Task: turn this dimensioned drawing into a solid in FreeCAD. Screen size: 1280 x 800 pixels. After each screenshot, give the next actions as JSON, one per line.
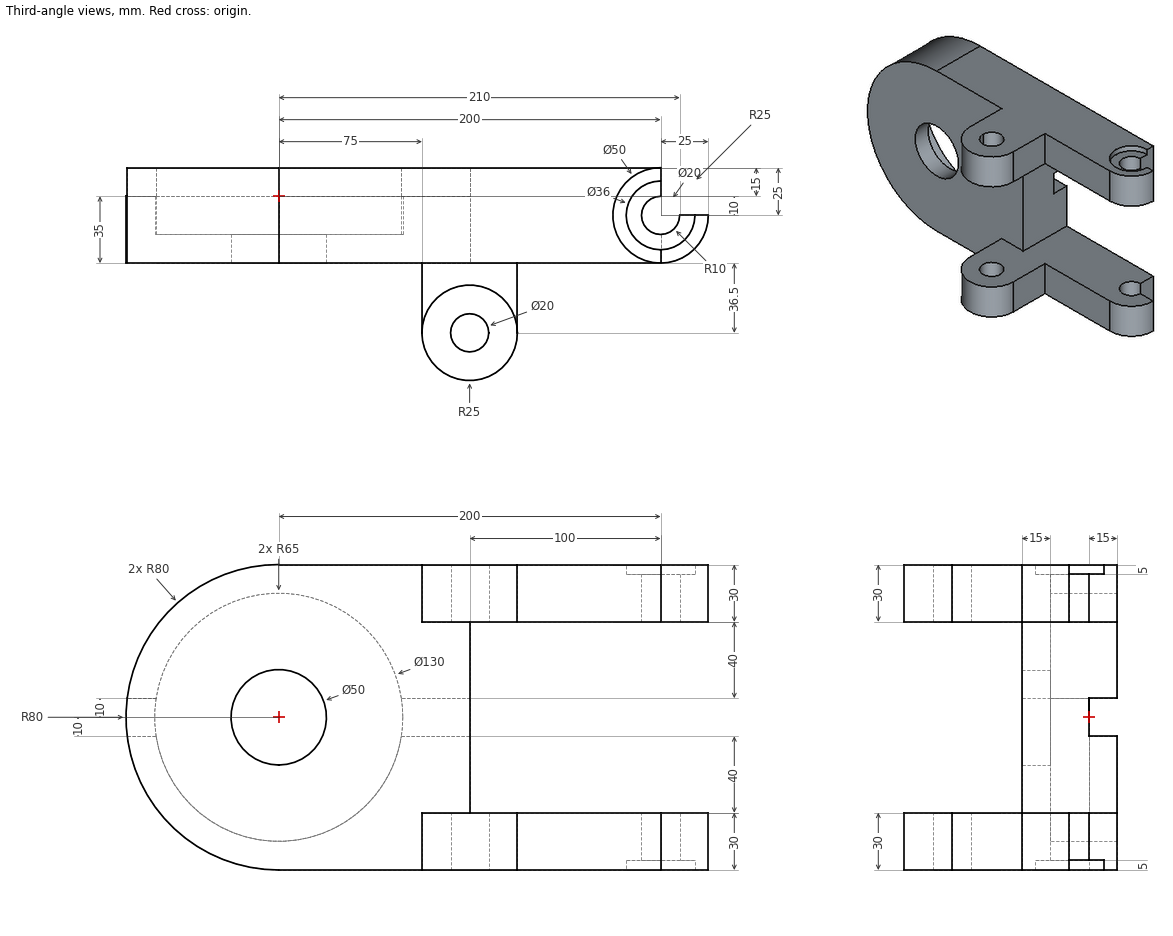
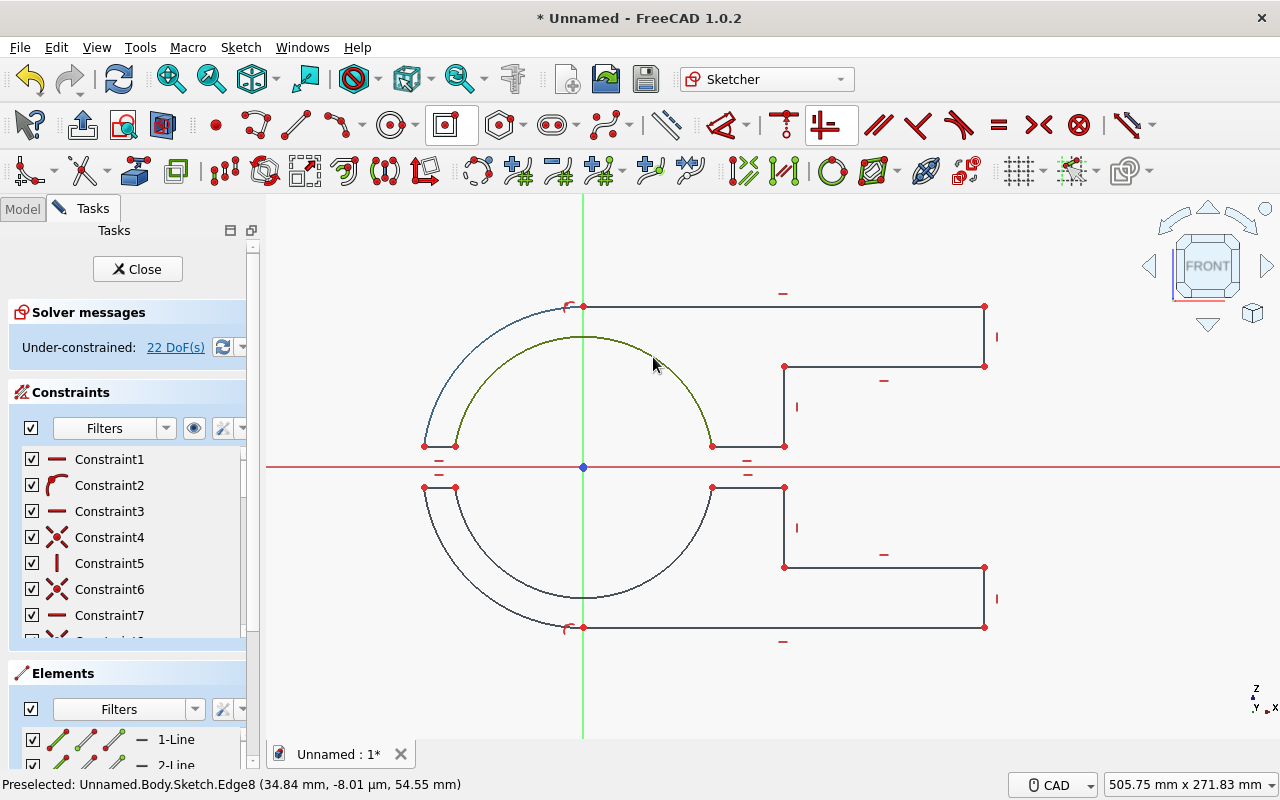
{"action": "left_click", "coordinate": [784, 126]}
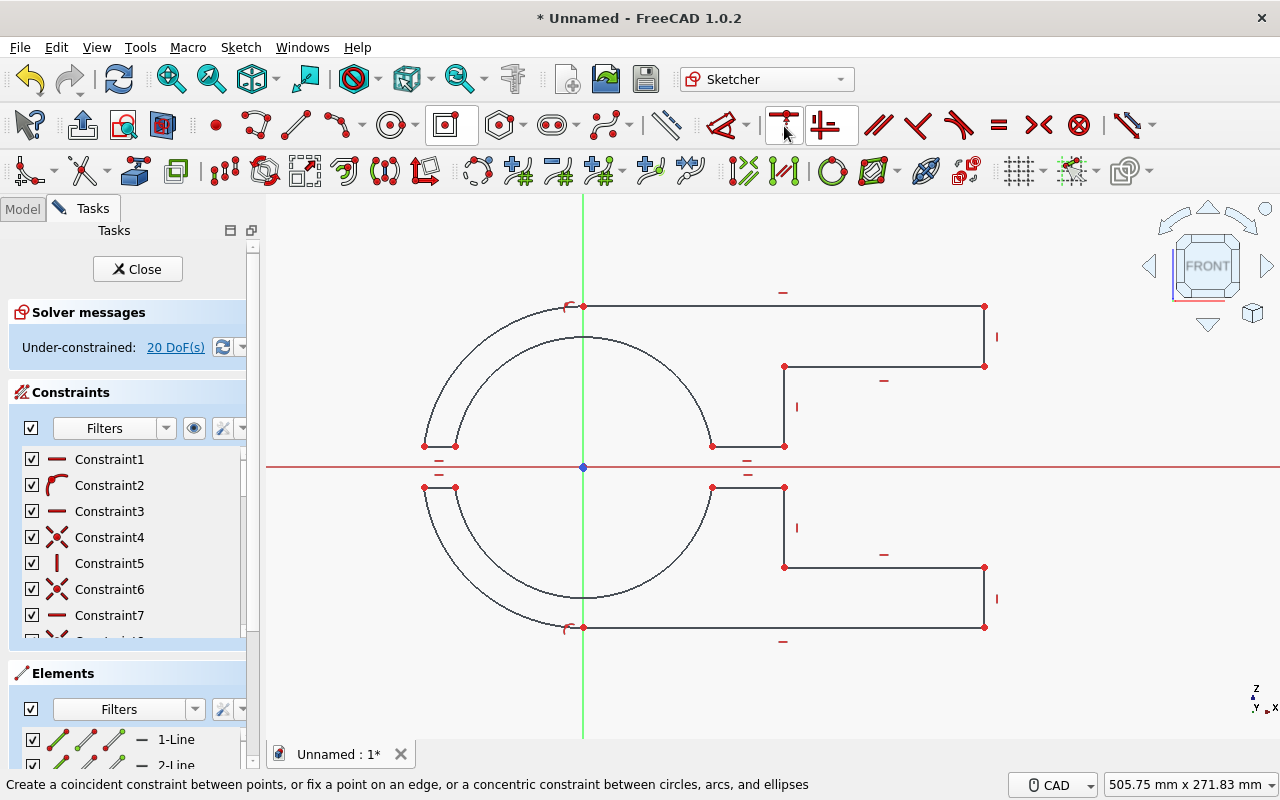
{"action": "left_click", "coordinate": [516, 321]}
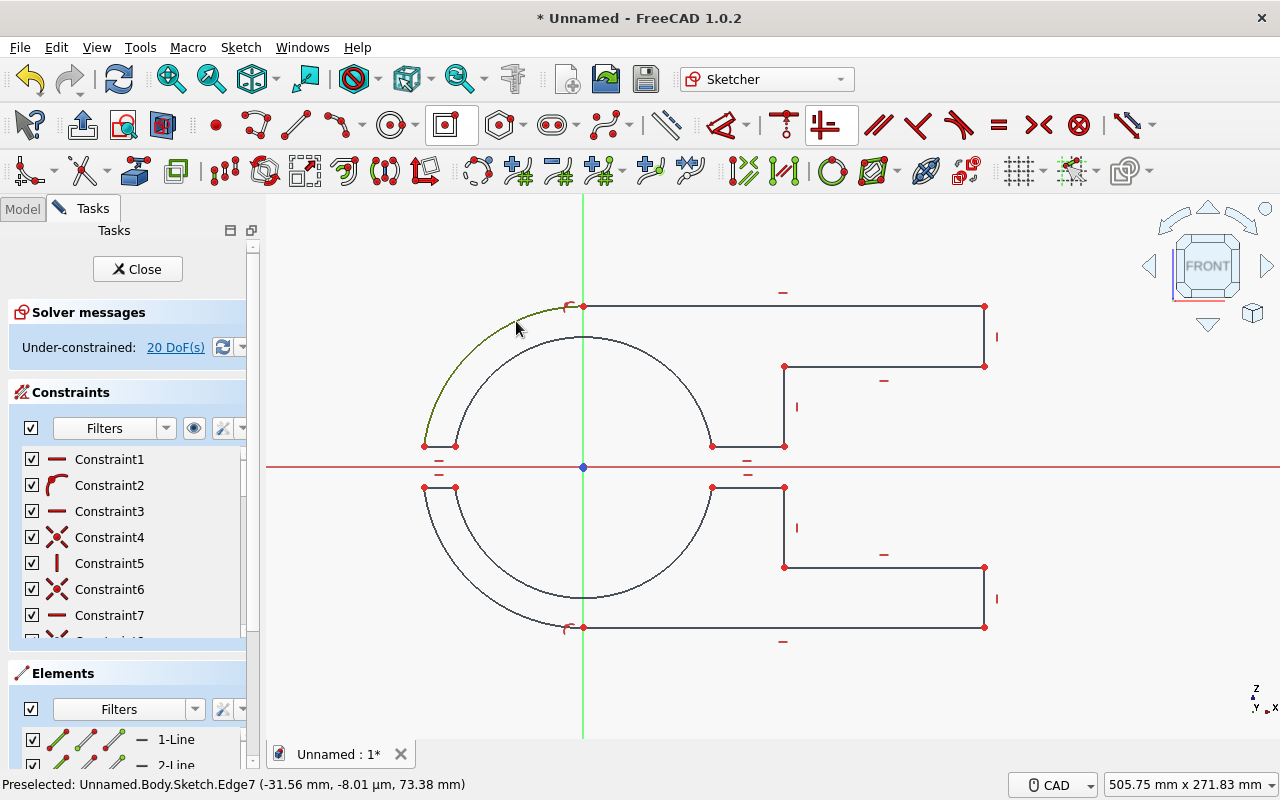
{"action": "left_click", "coordinate": [514, 578]}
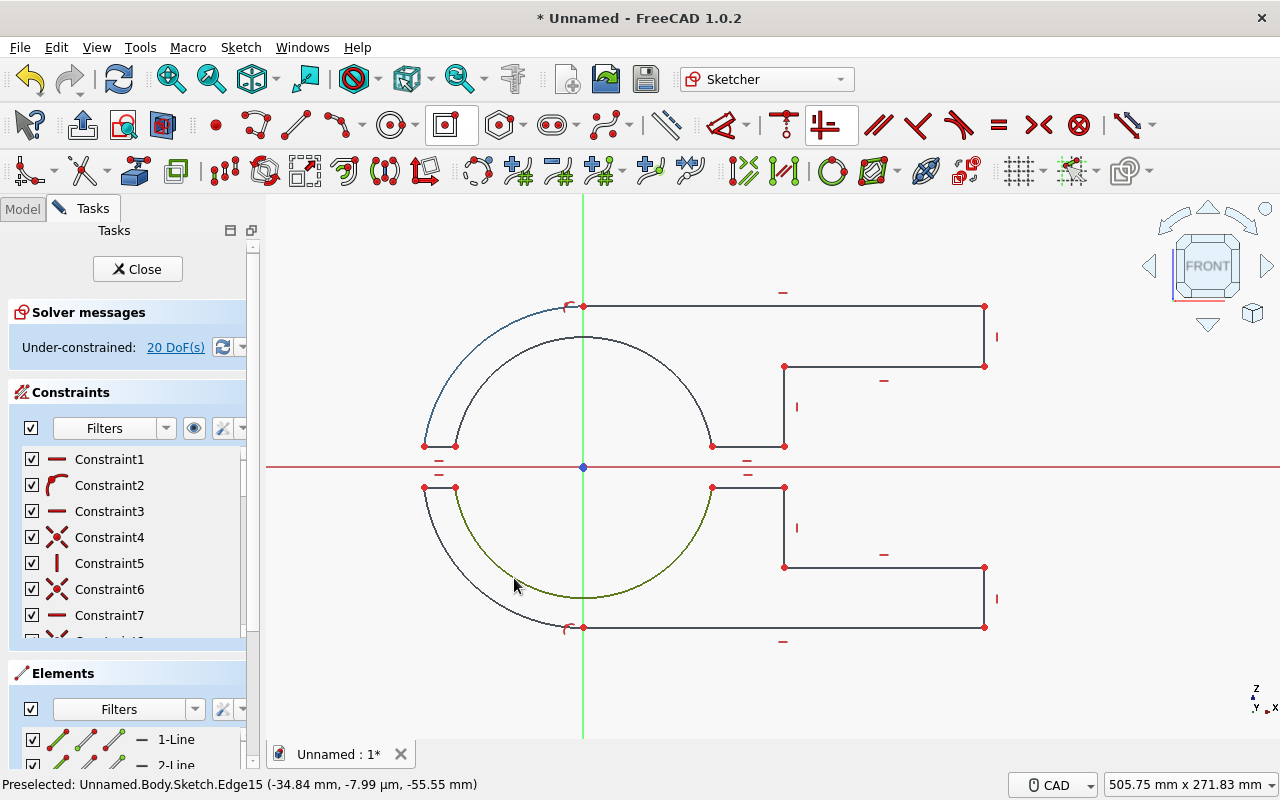
{"action": "left_click", "coordinate": [784, 126]}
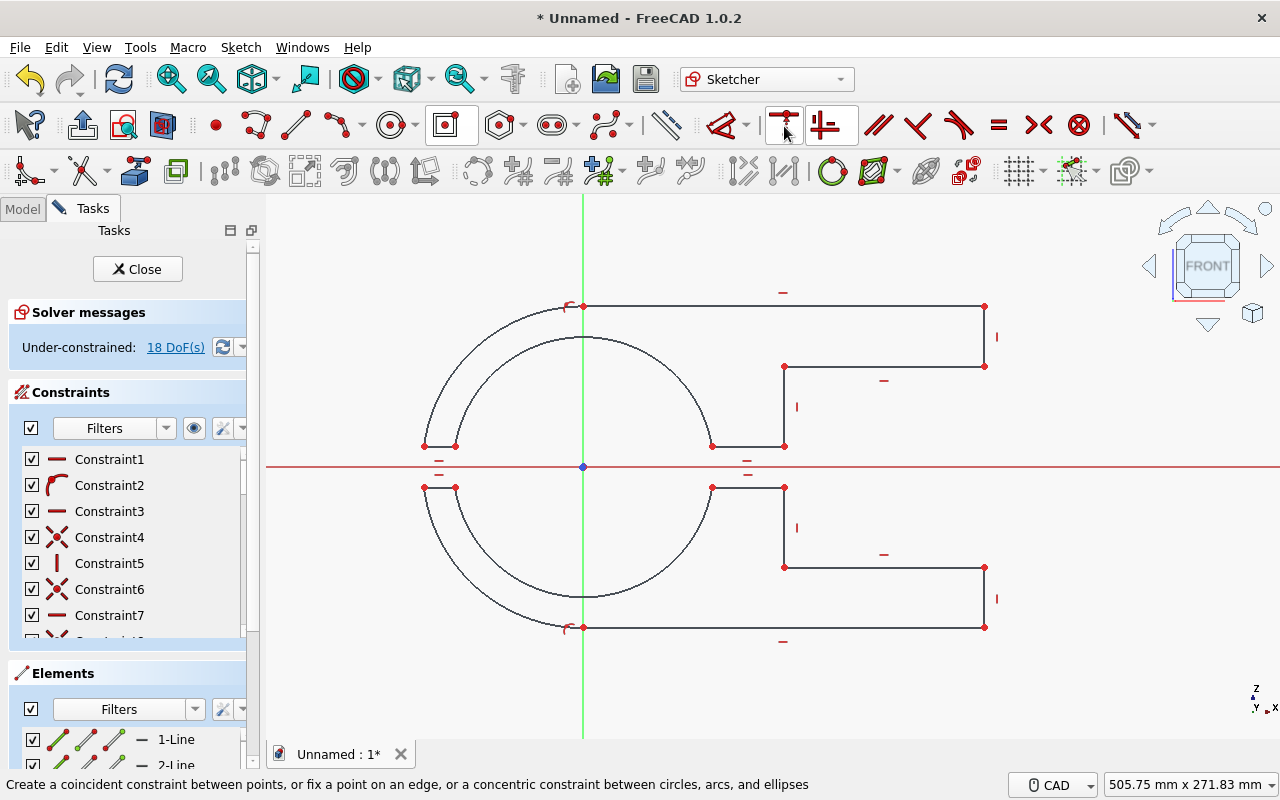
{"action": "left_click", "coordinate": [516, 321]}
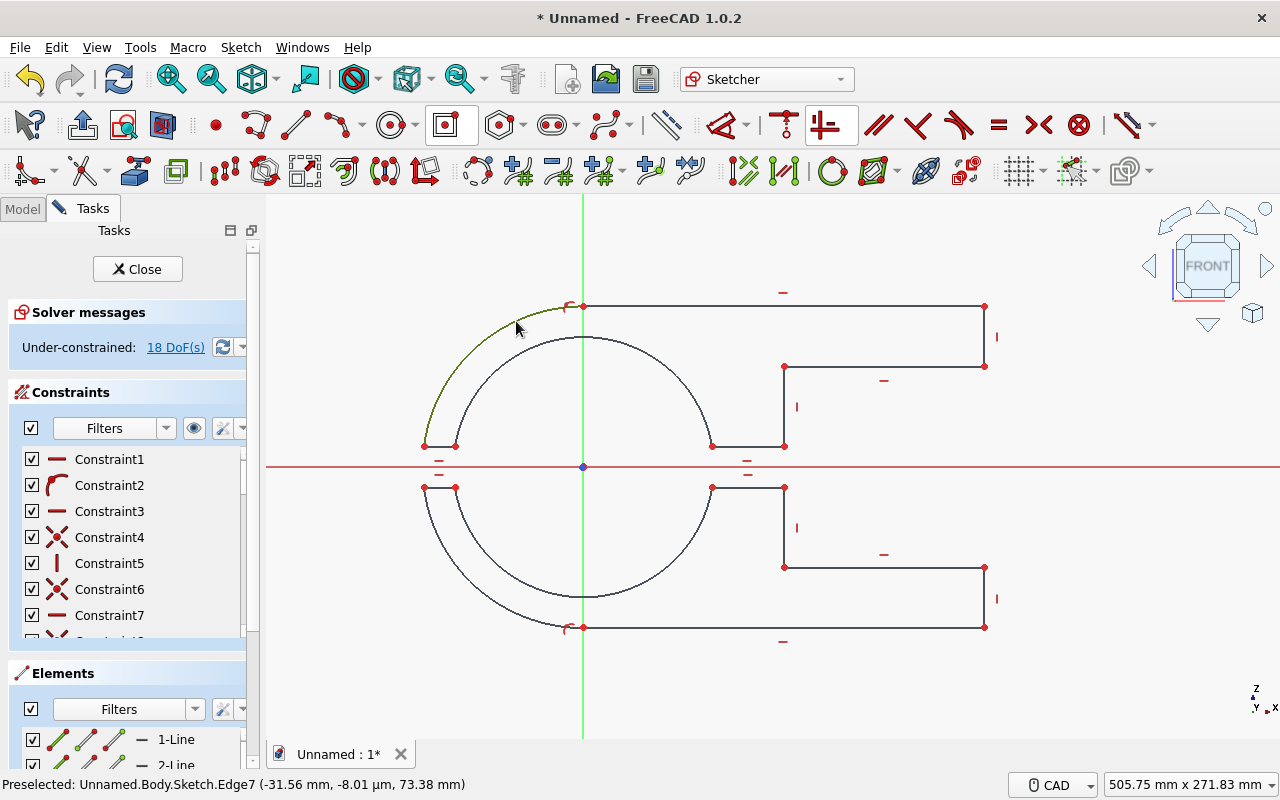
{"action": "left_click", "coordinate": [447, 553]}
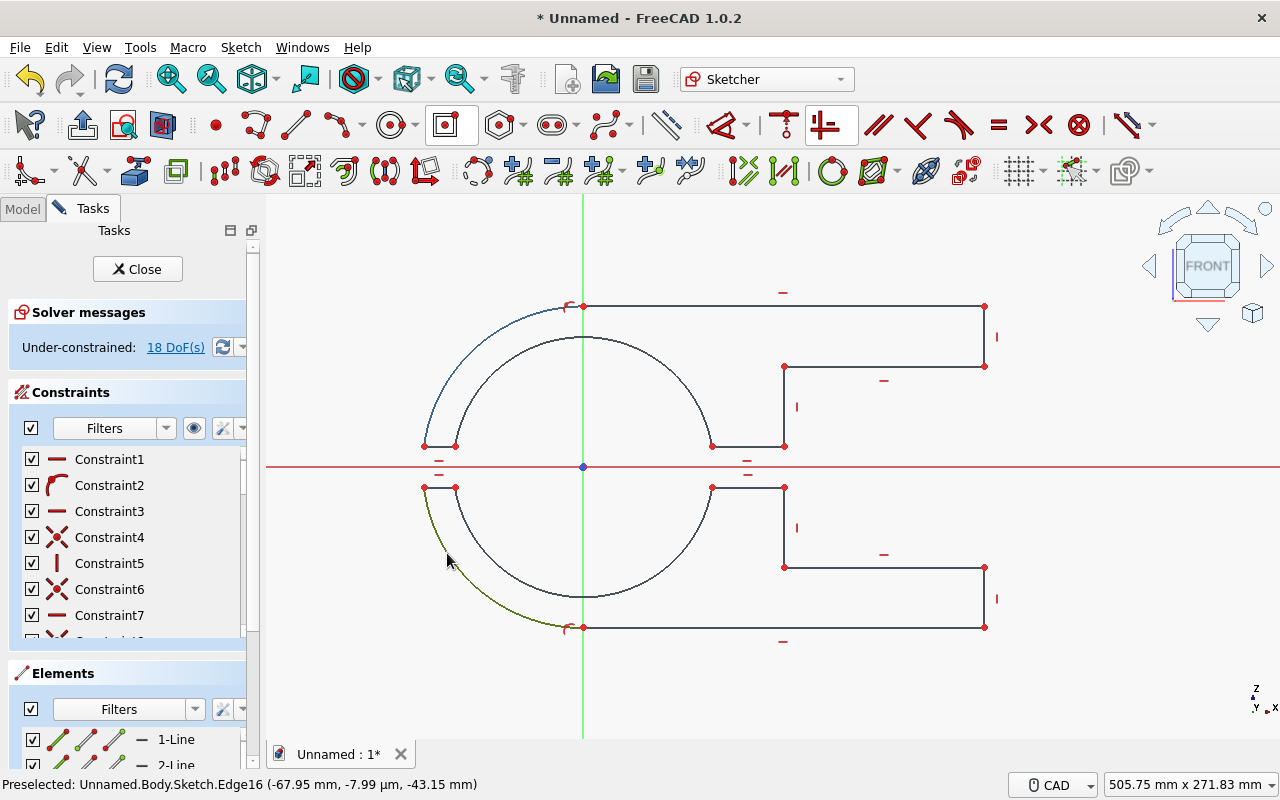
{"action": "left_click", "coordinate": [784, 126]}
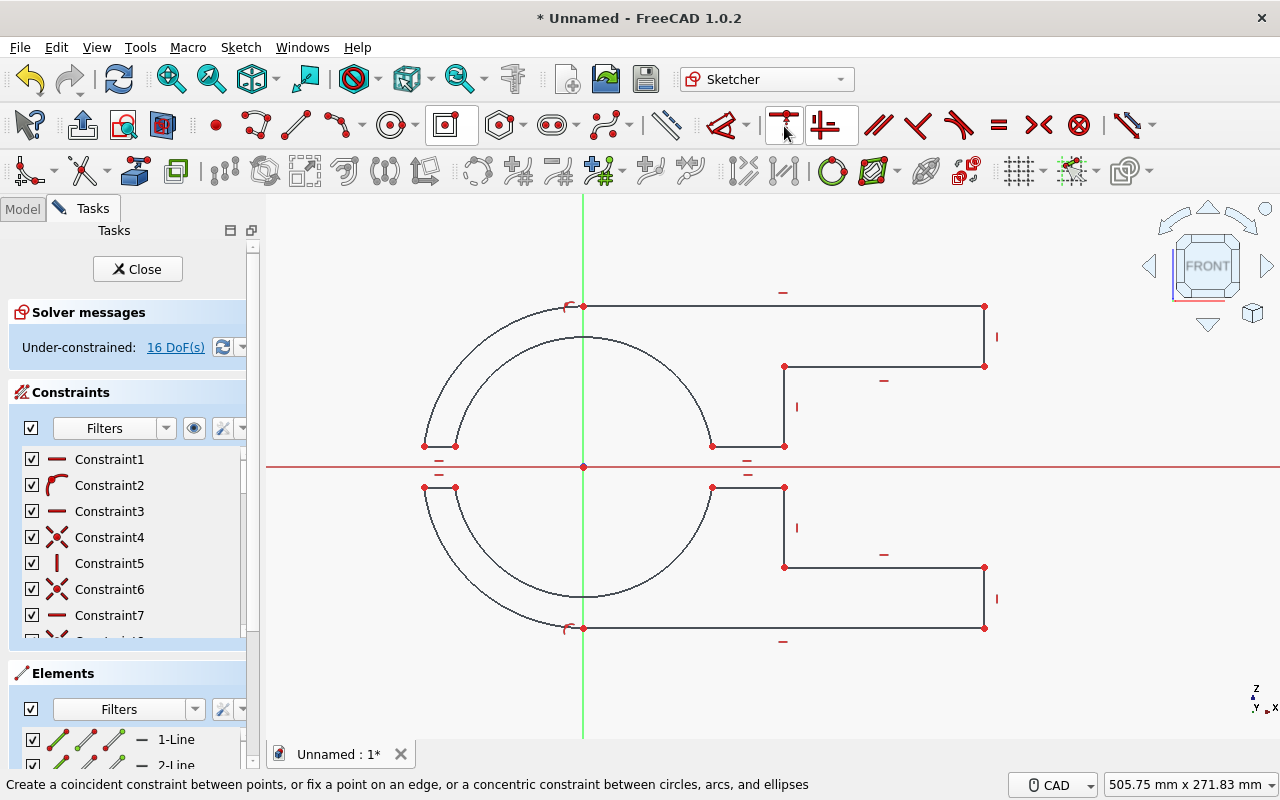
{"action": "left_click_drag", "start_coordinate": [573, 456], "coordinate": [593, 477]}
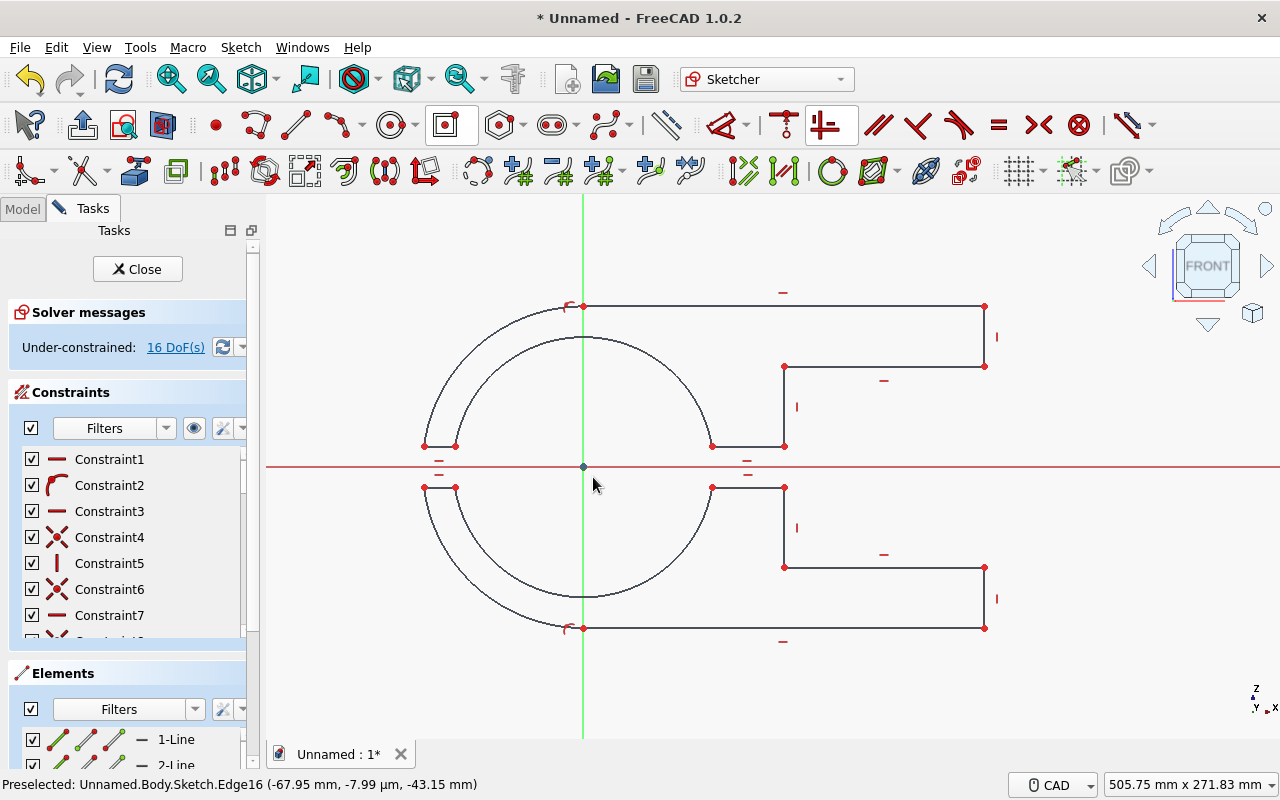
{"action": "left_click", "coordinate": [784, 126]}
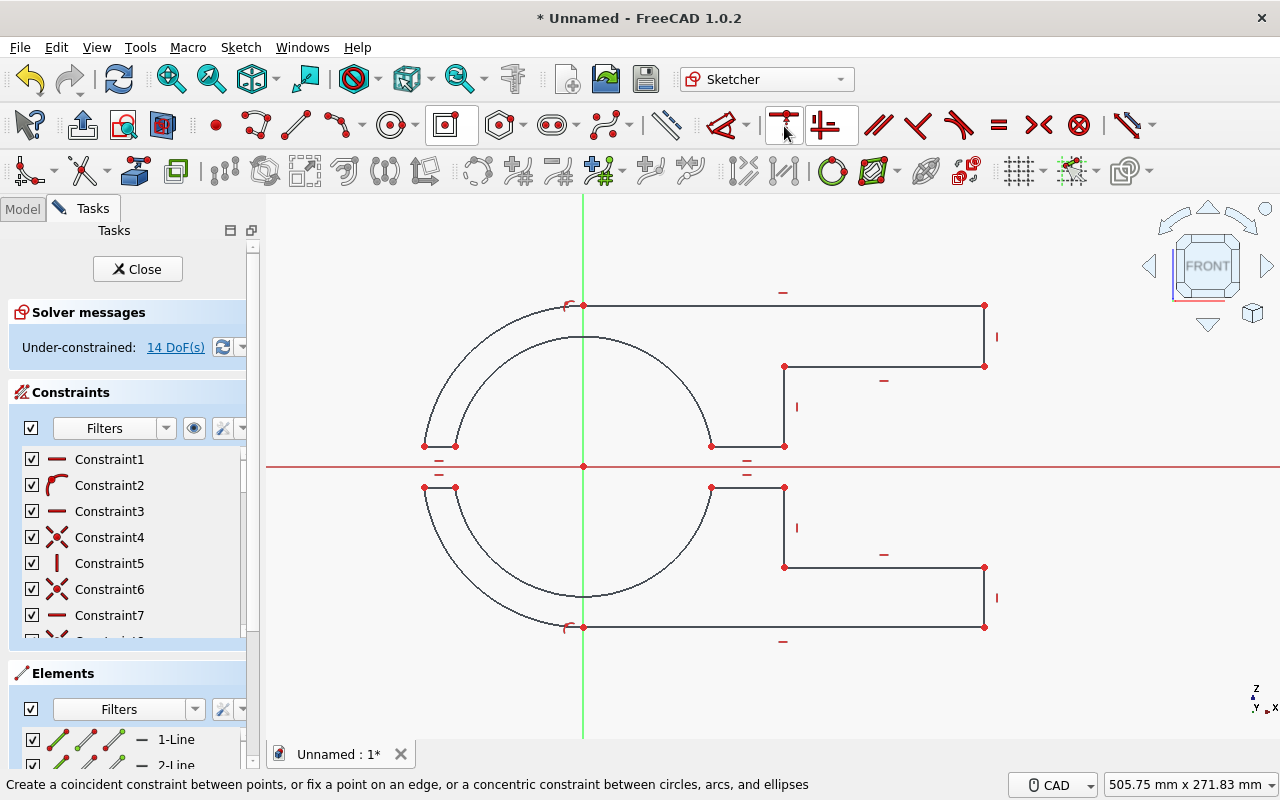
{"action": "left_click", "coordinate": [653, 357]}